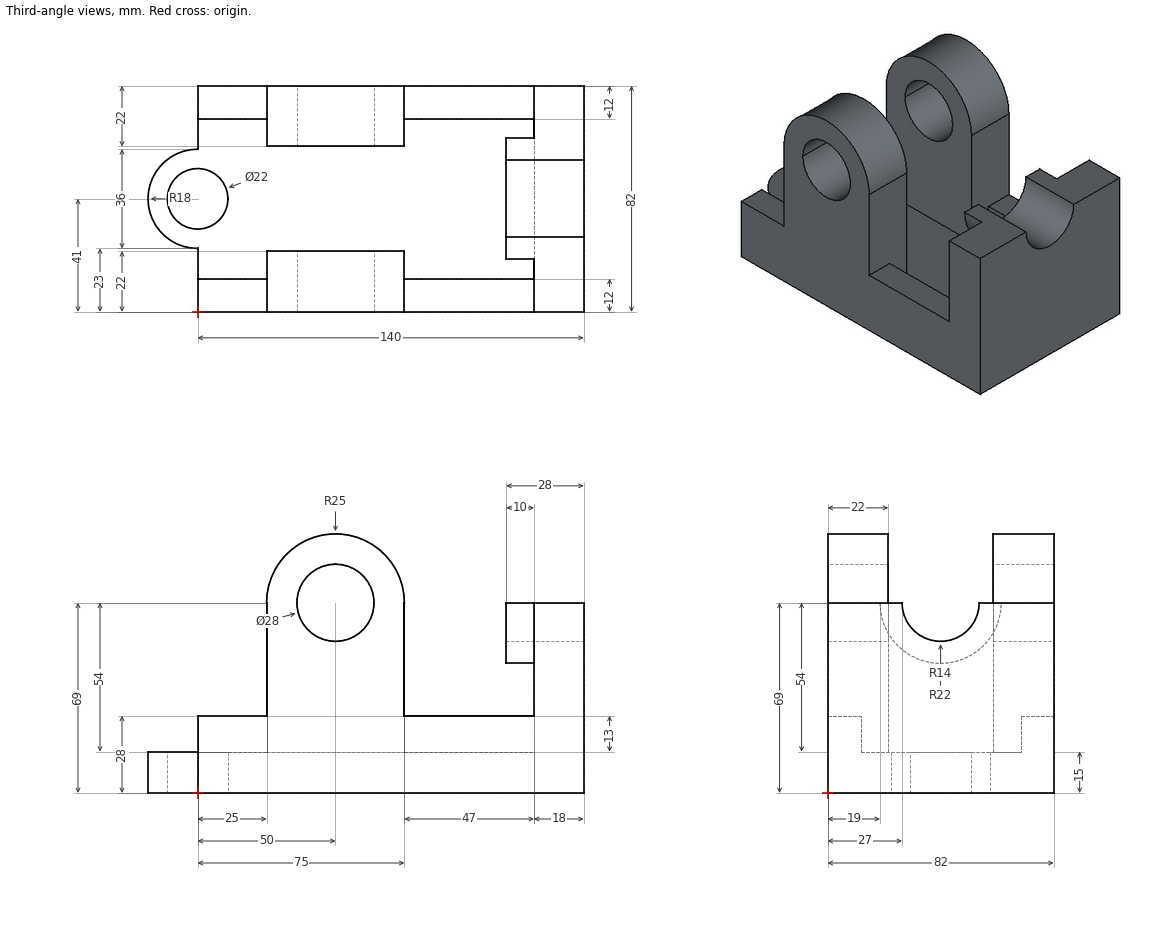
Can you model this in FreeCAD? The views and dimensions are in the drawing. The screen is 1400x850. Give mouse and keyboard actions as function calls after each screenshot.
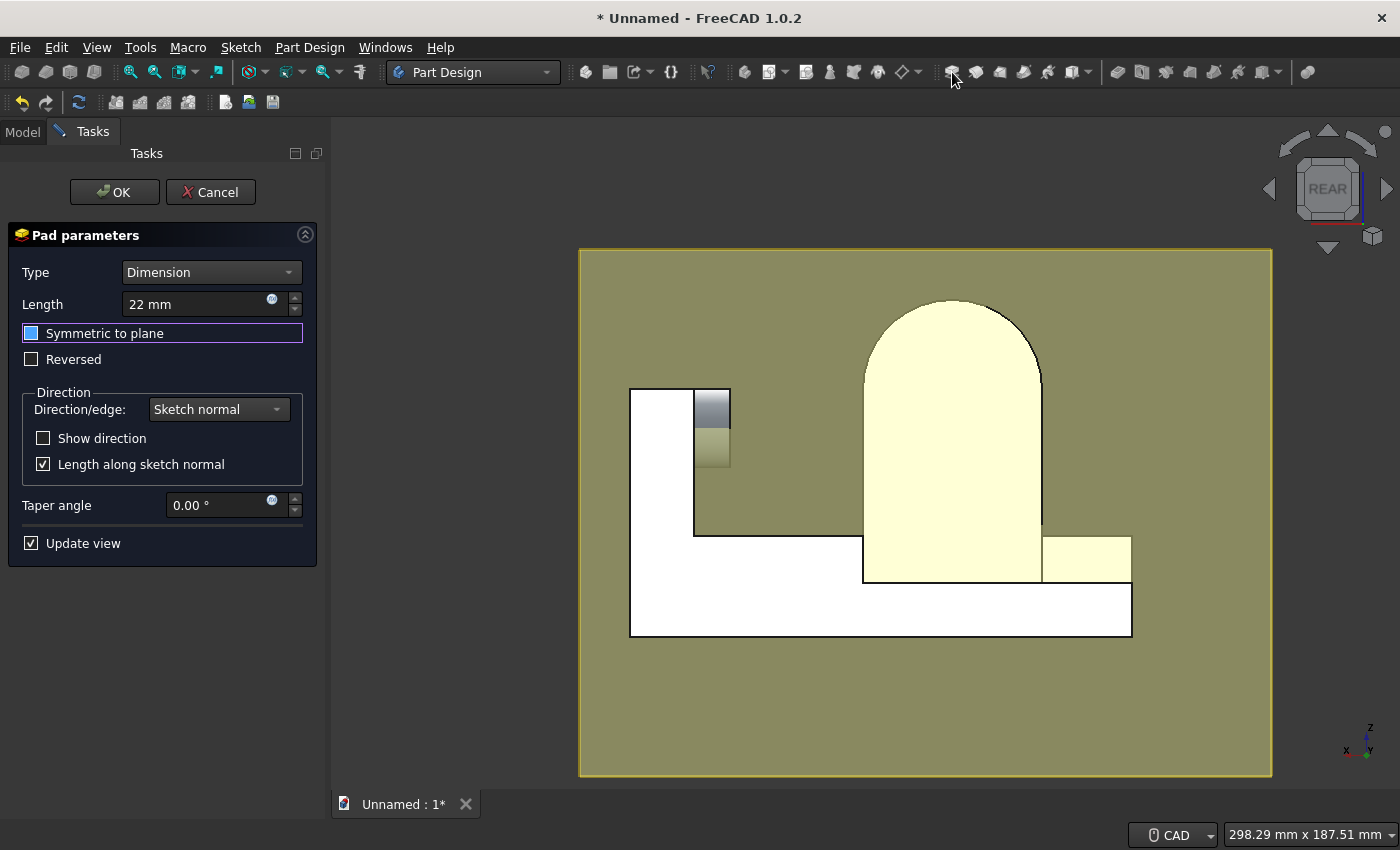
click(30, 359)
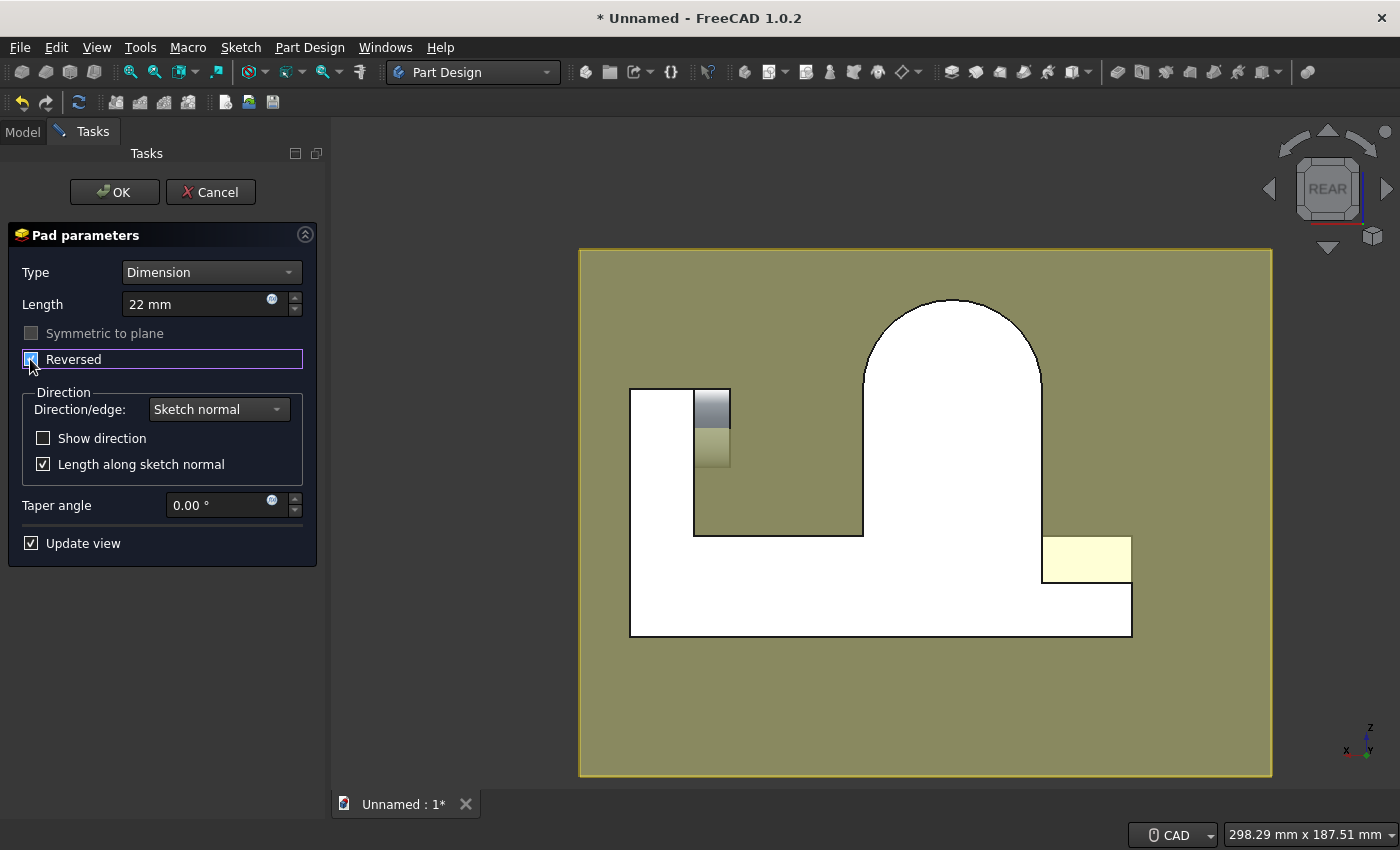
click(115, 192)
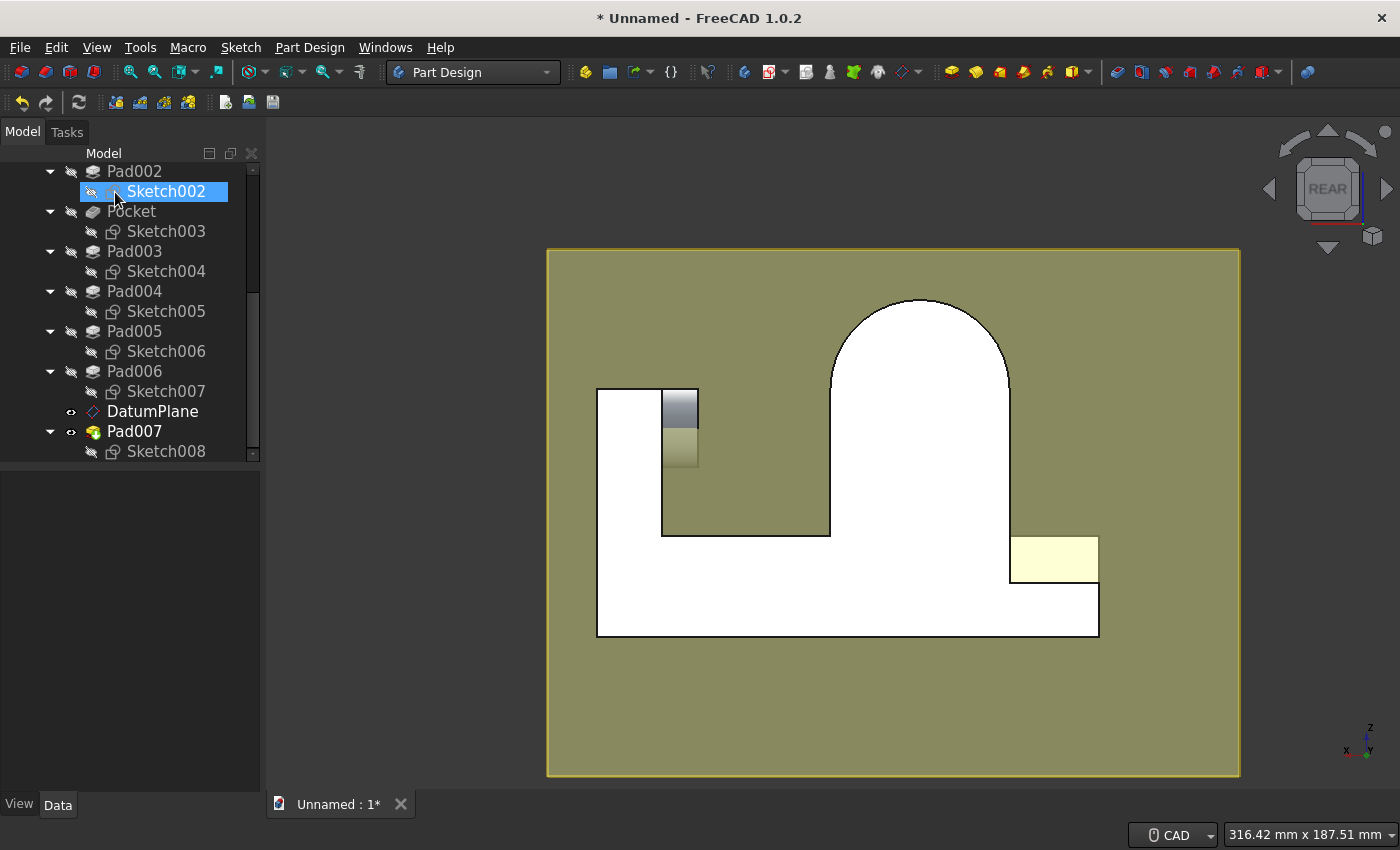
click(116, 412)
key(space)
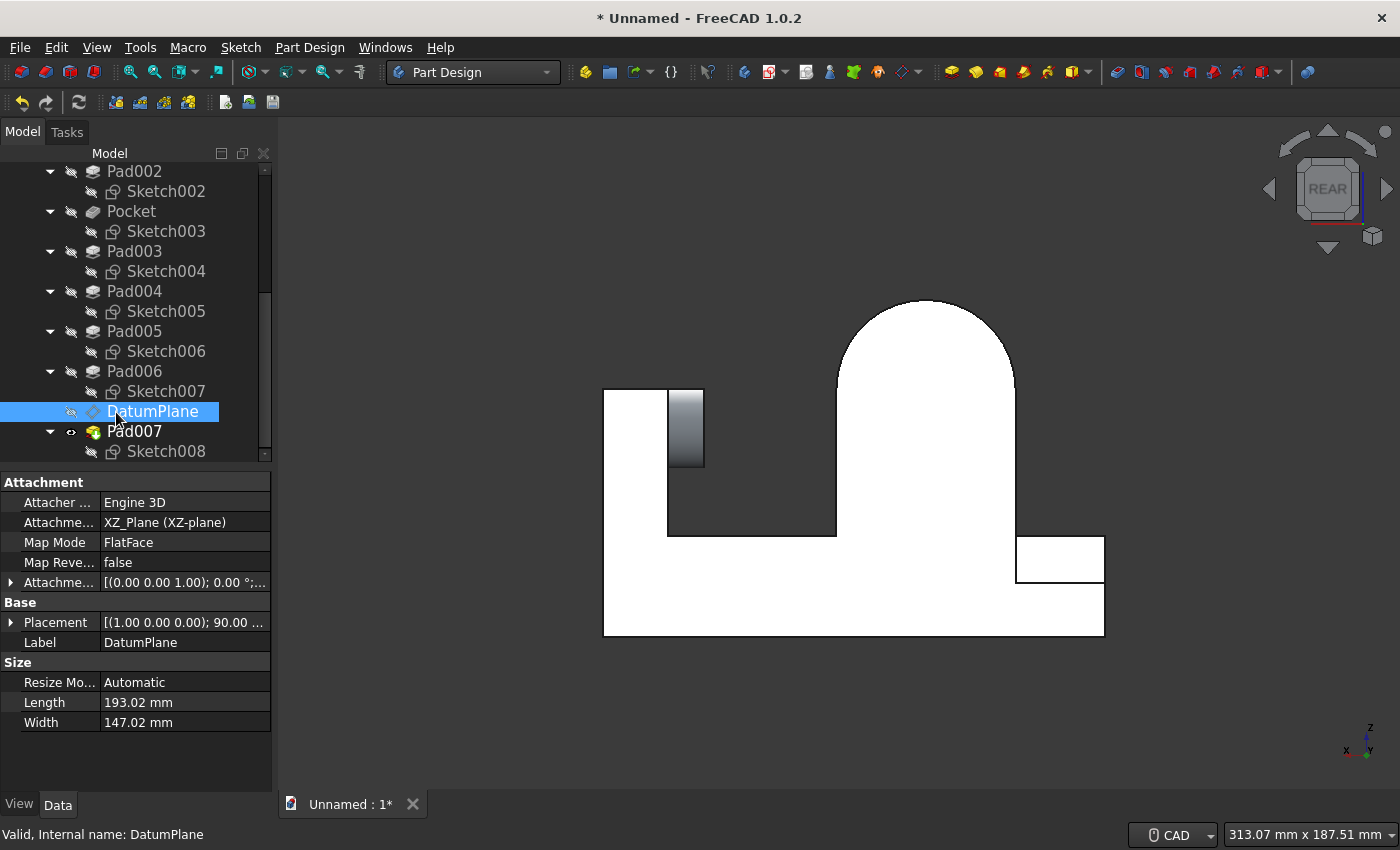
click(926, 419)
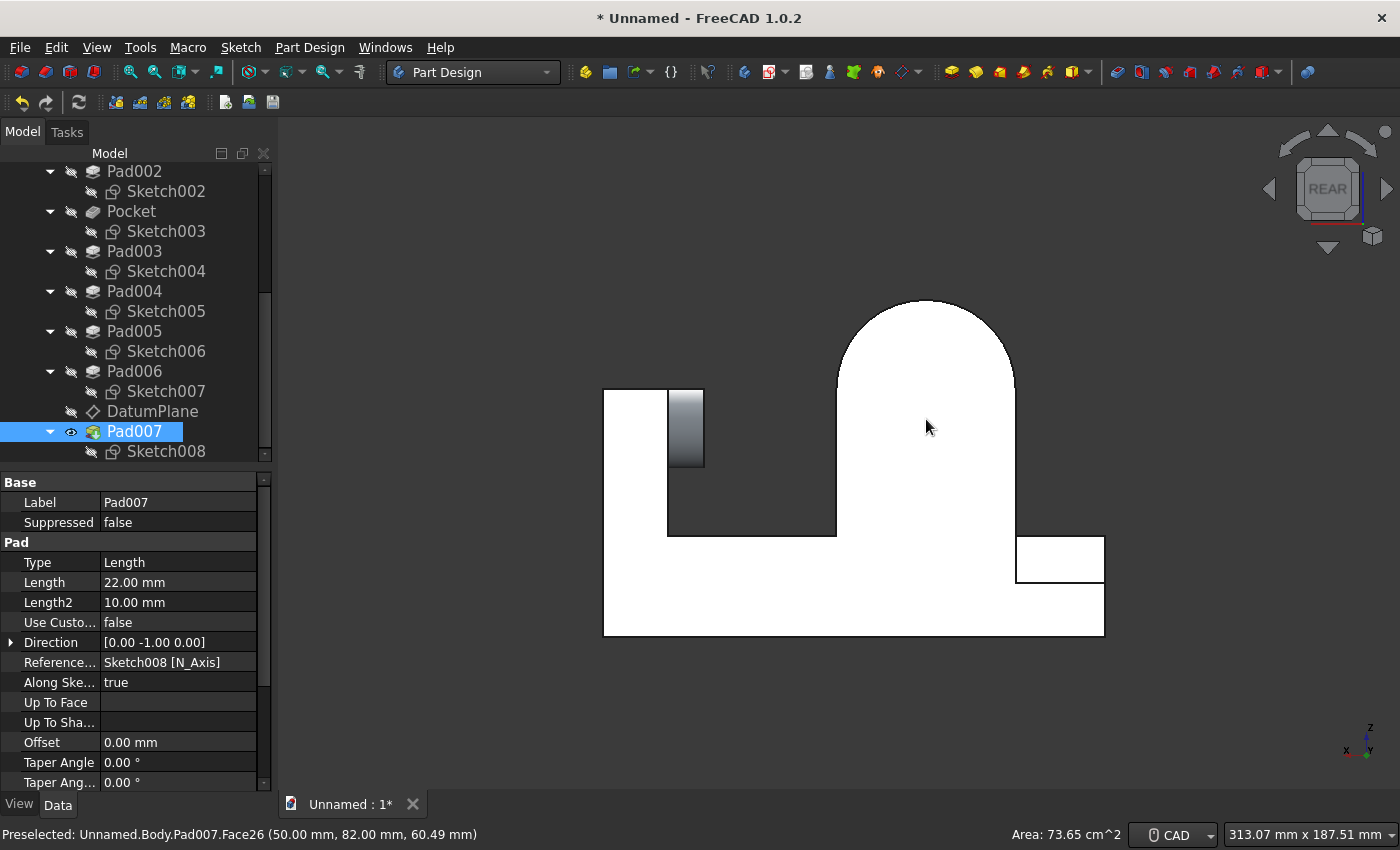
click(770, 72)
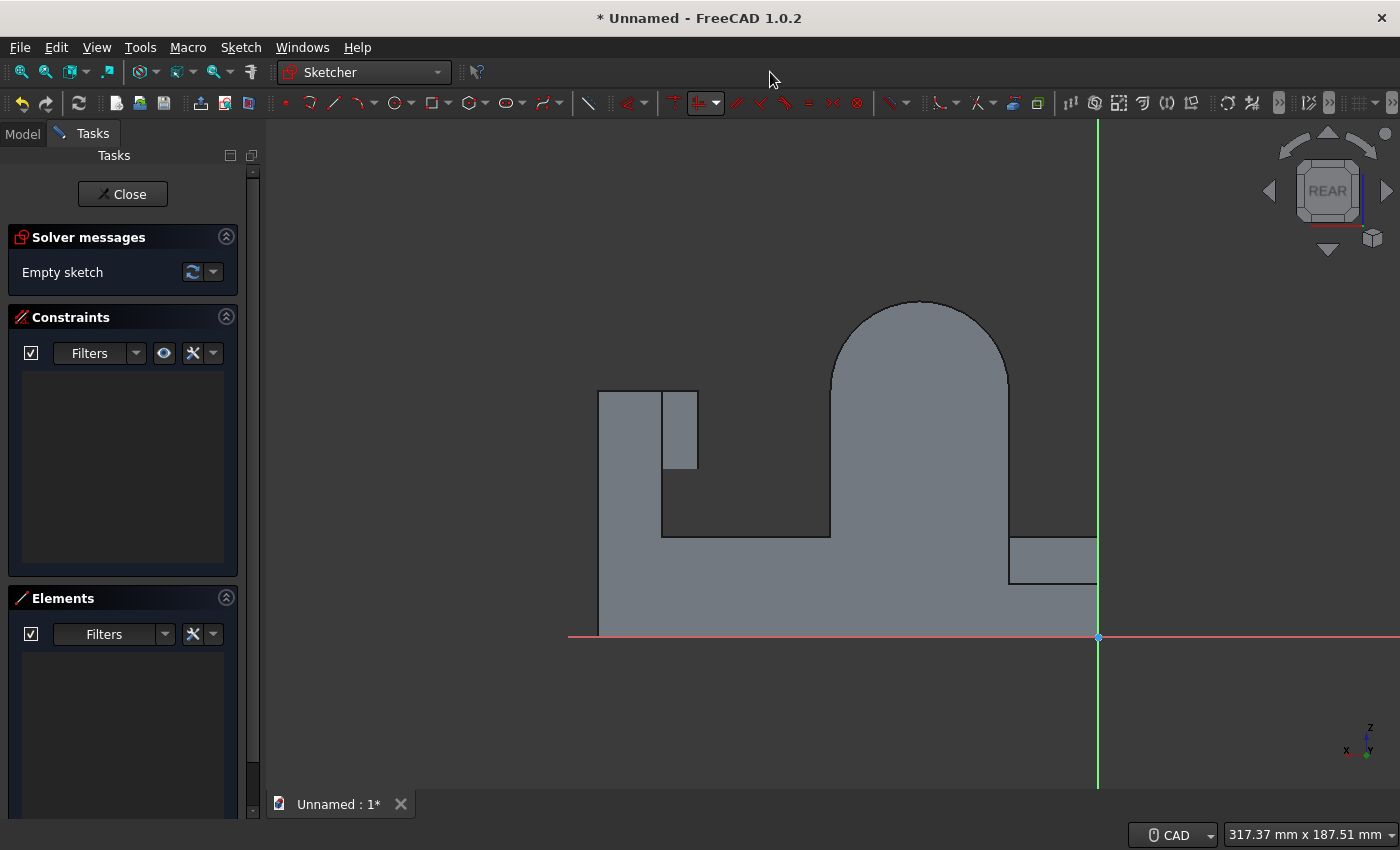
scroll(1148, 631, up, 7)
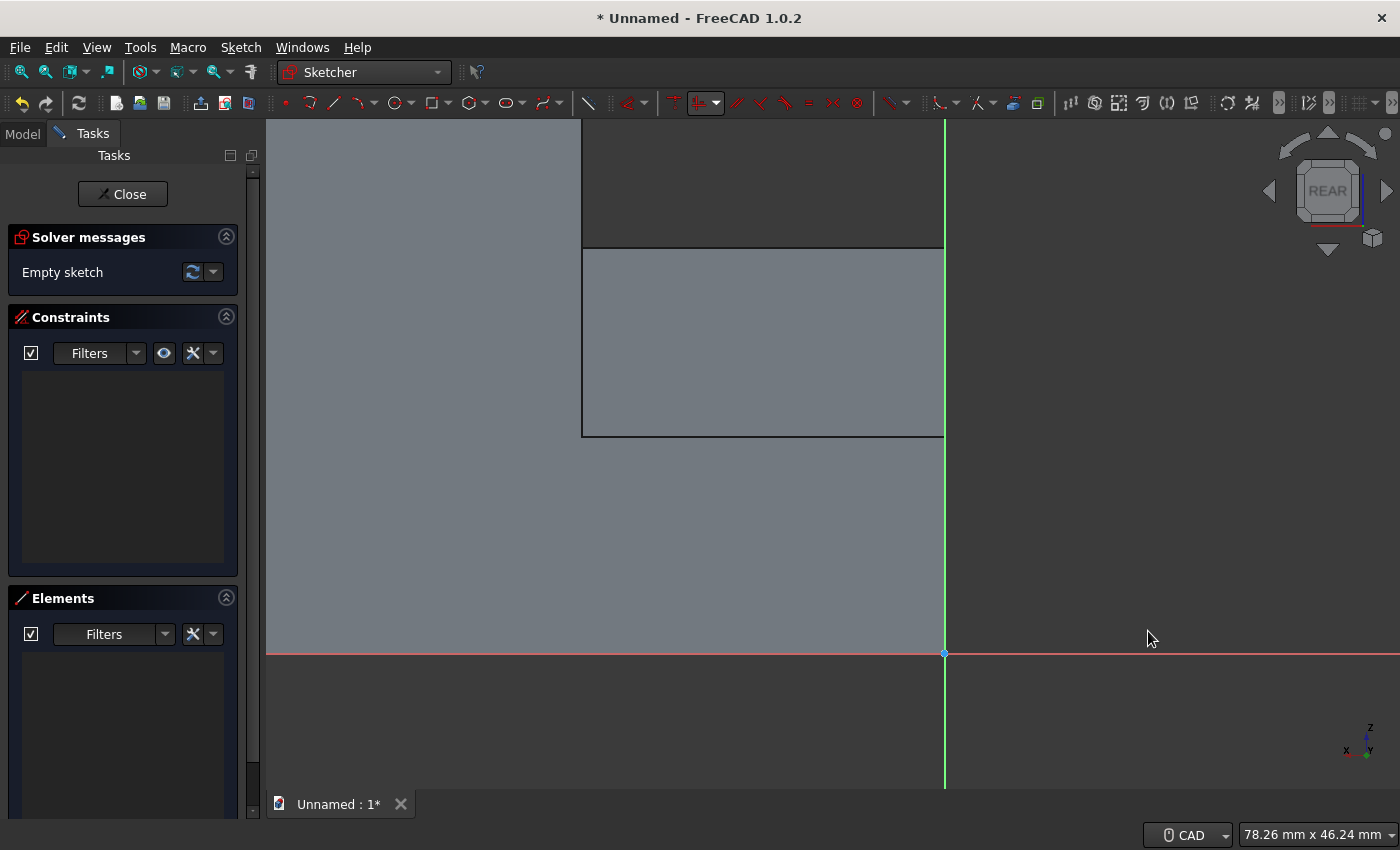
click(432, 104)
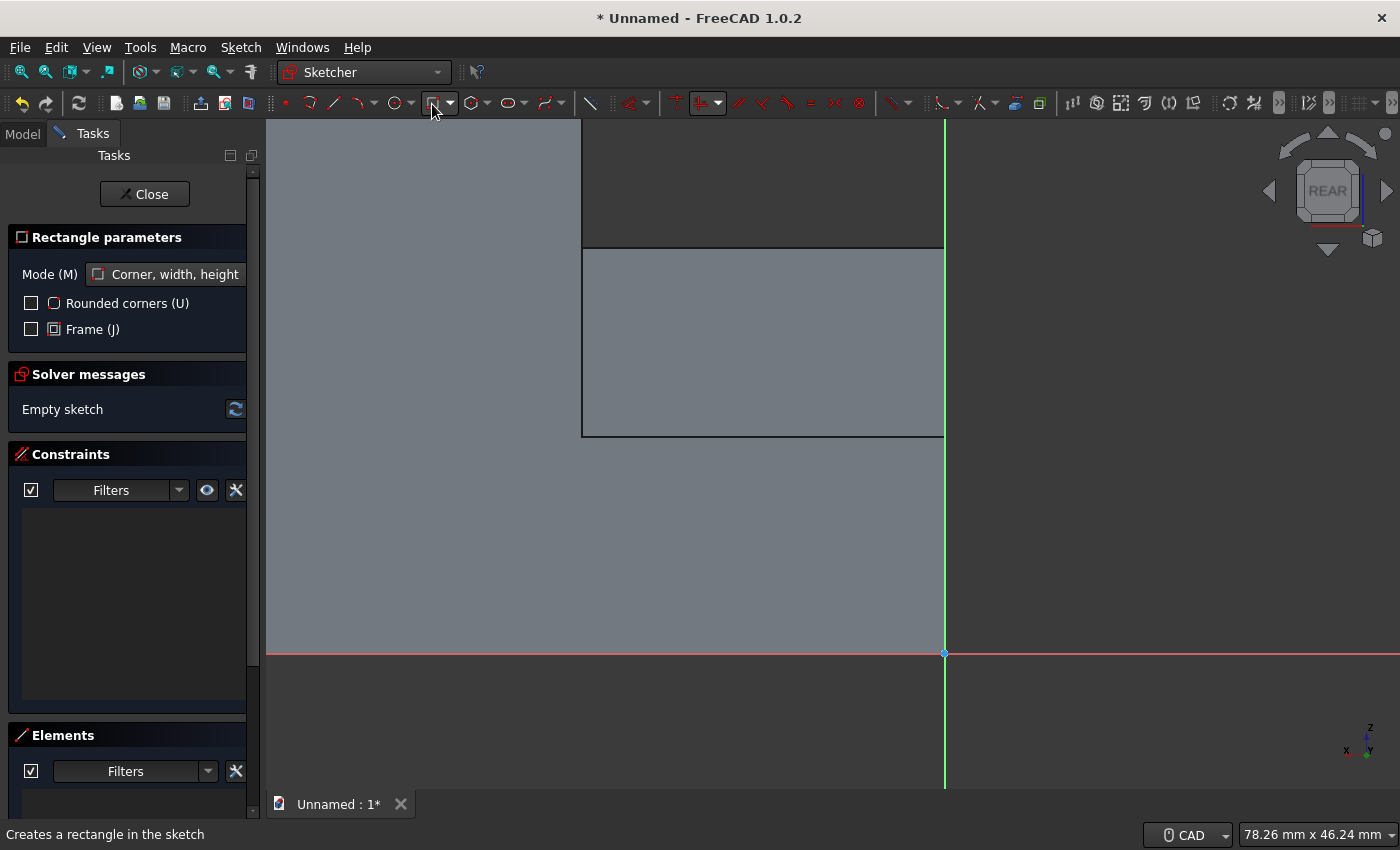
click(582, 248)
click(945, 437)
key(Escape)